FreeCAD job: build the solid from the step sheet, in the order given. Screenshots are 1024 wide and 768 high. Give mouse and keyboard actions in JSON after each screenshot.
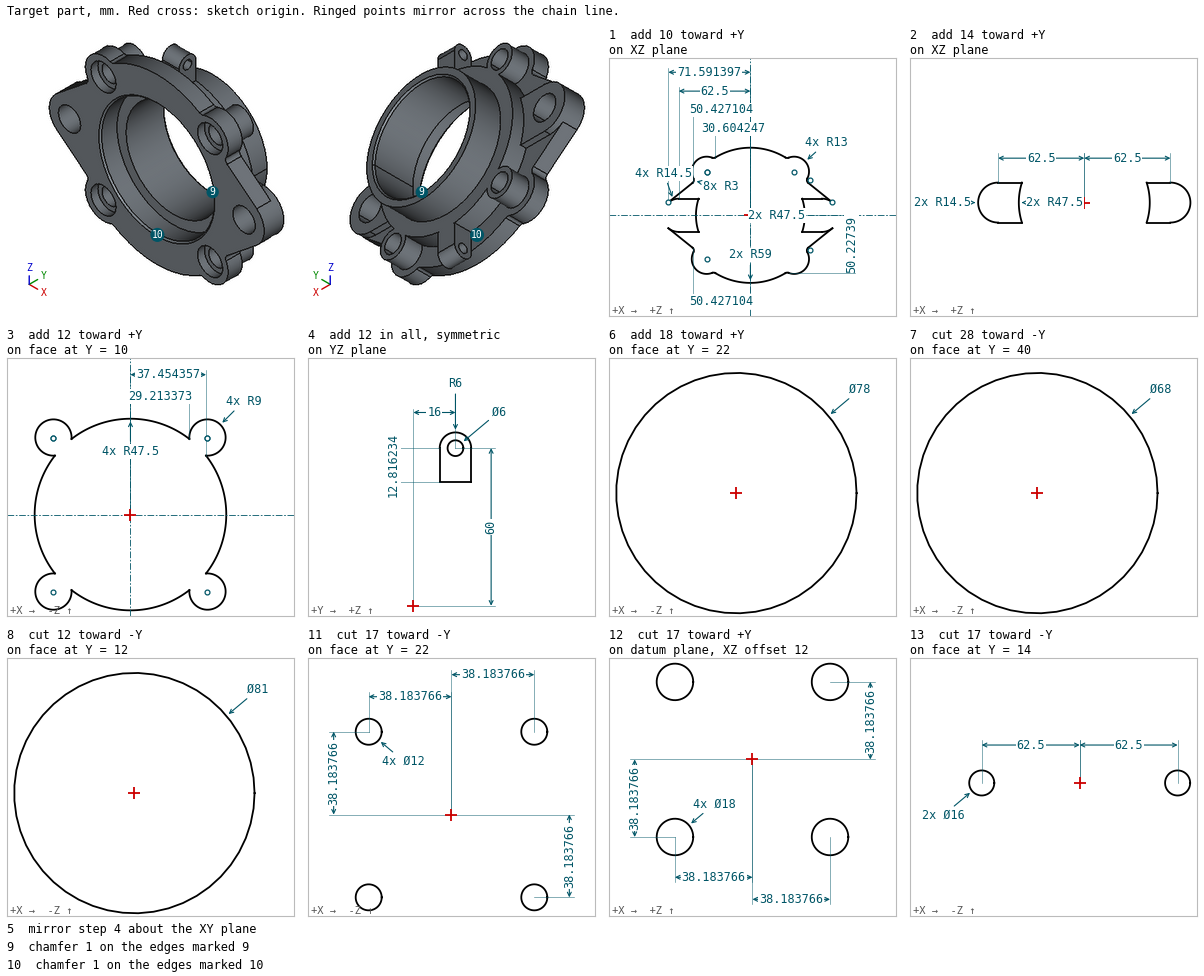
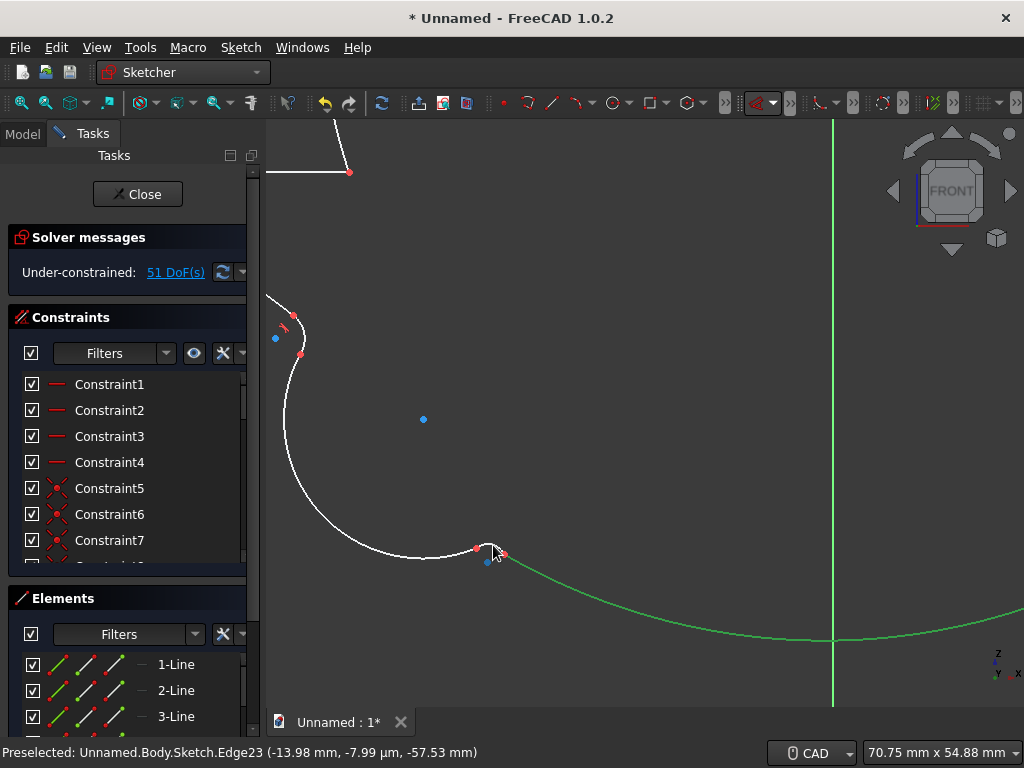
{"action": "left_click", "coordinate": [492, 545]}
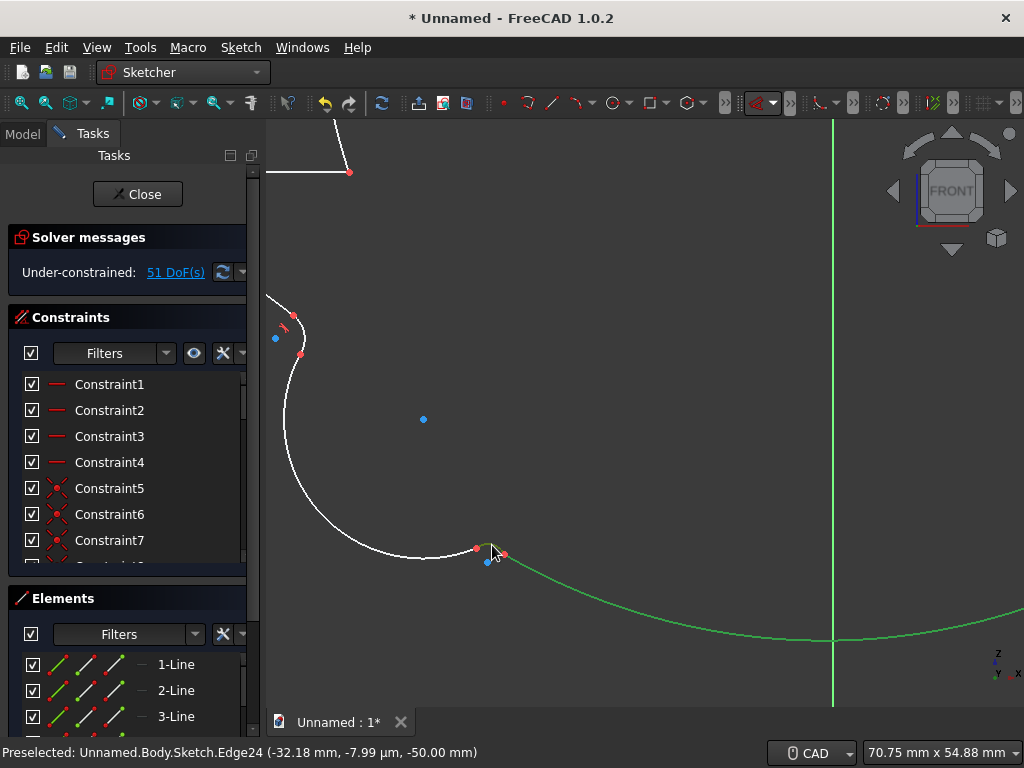
{"action": "key", "text": "t"}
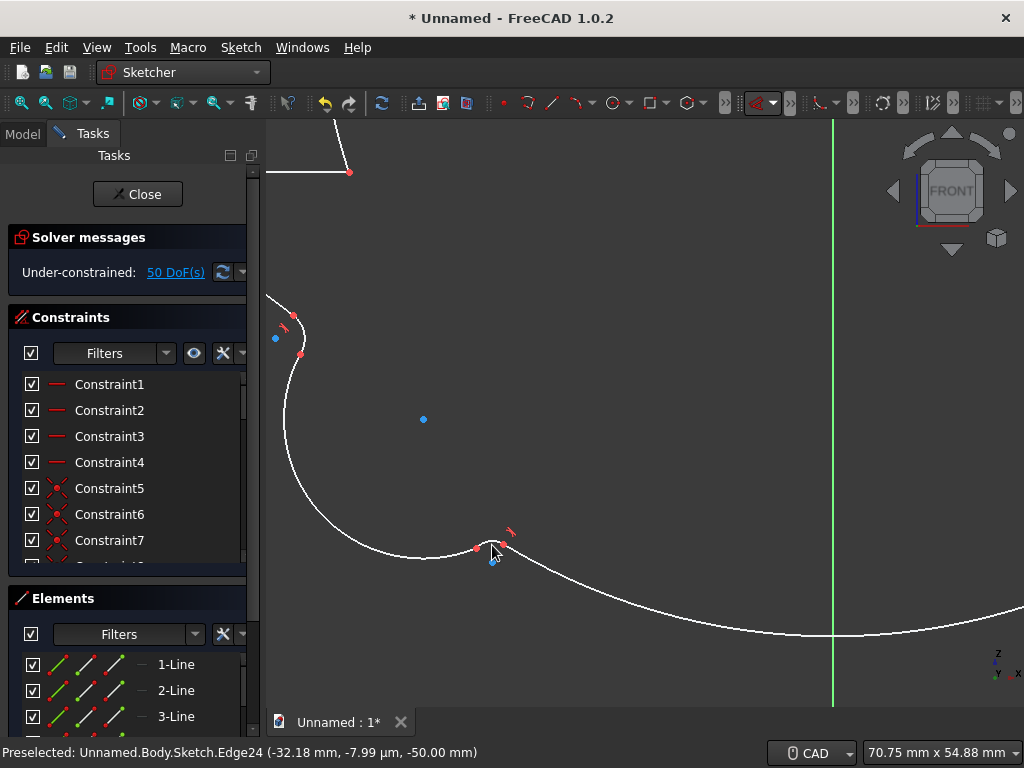
{"action": "left_click", "coordinate": [489, 541]}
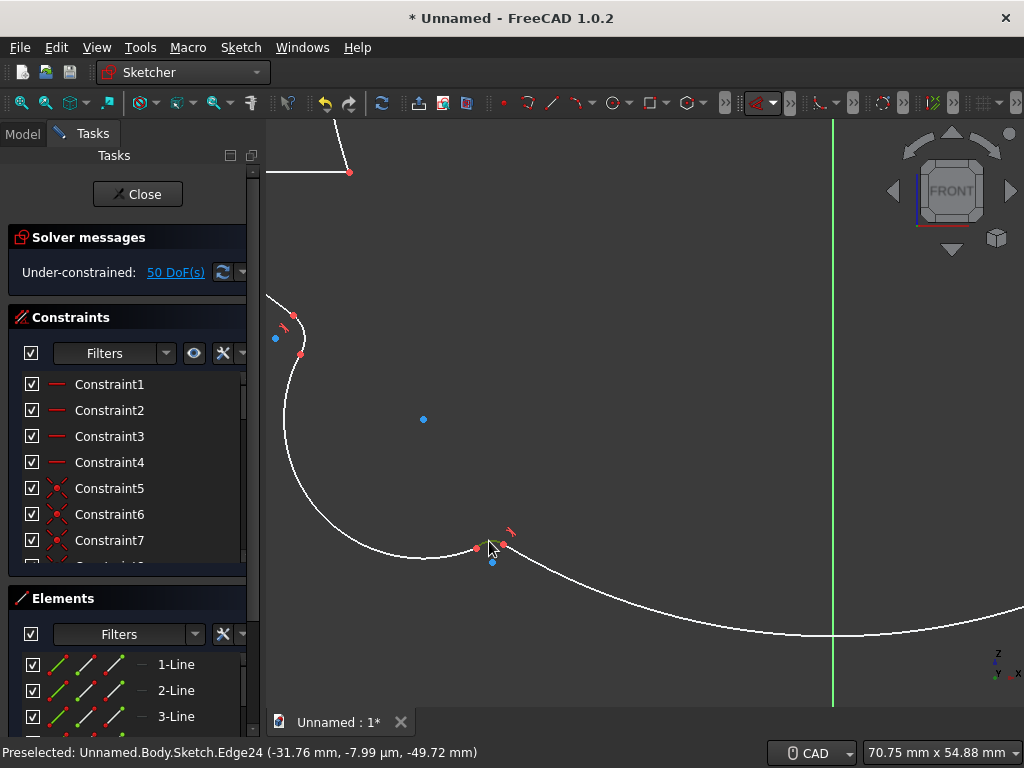
{"action": "scroll", "coordinate": [493, 545], "scroll_direction": "down", "scroll_amount": 7}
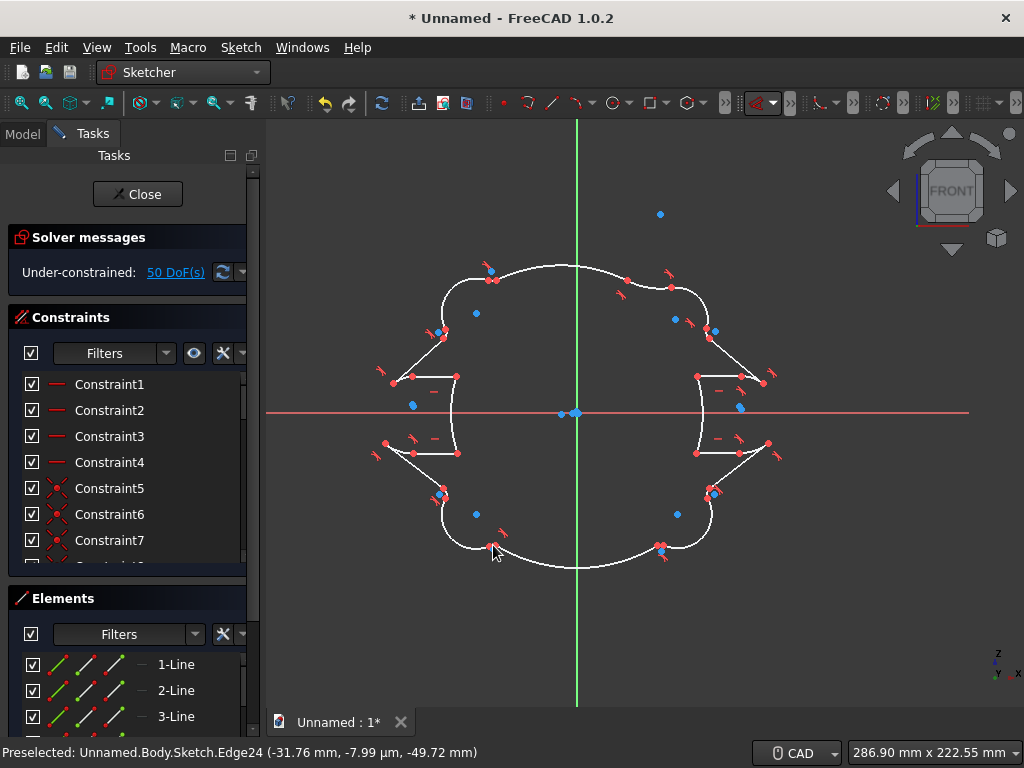
{"action": "left_click", "coordinate": [464, 547]}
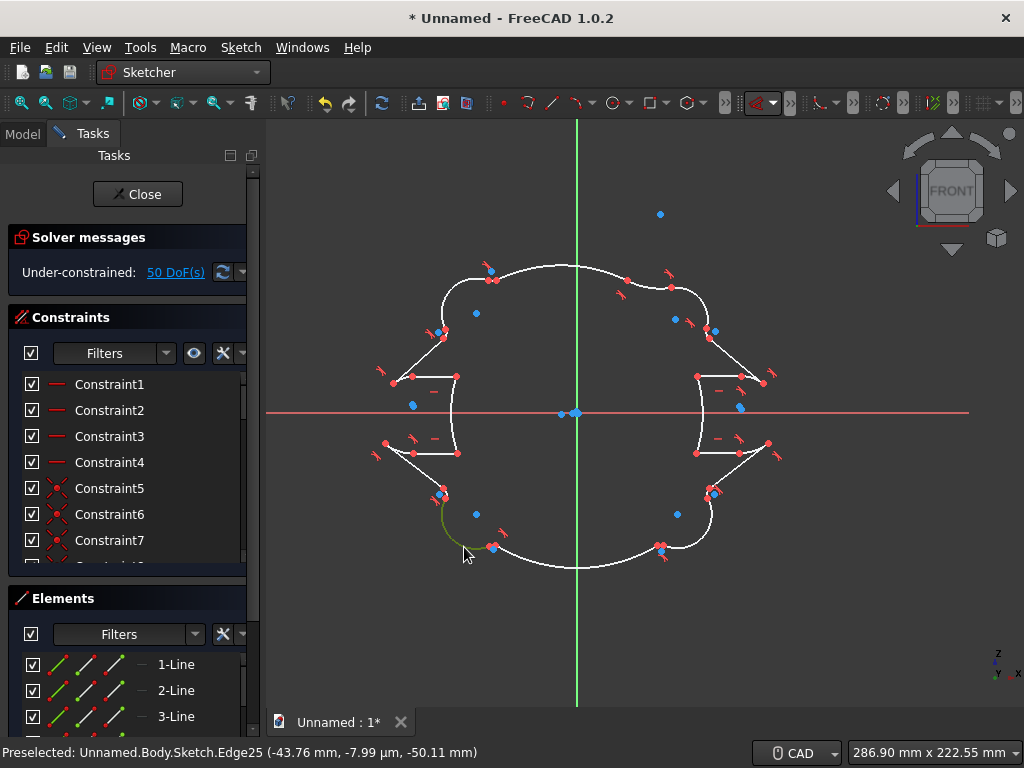
{"action": "key", "text": "t"}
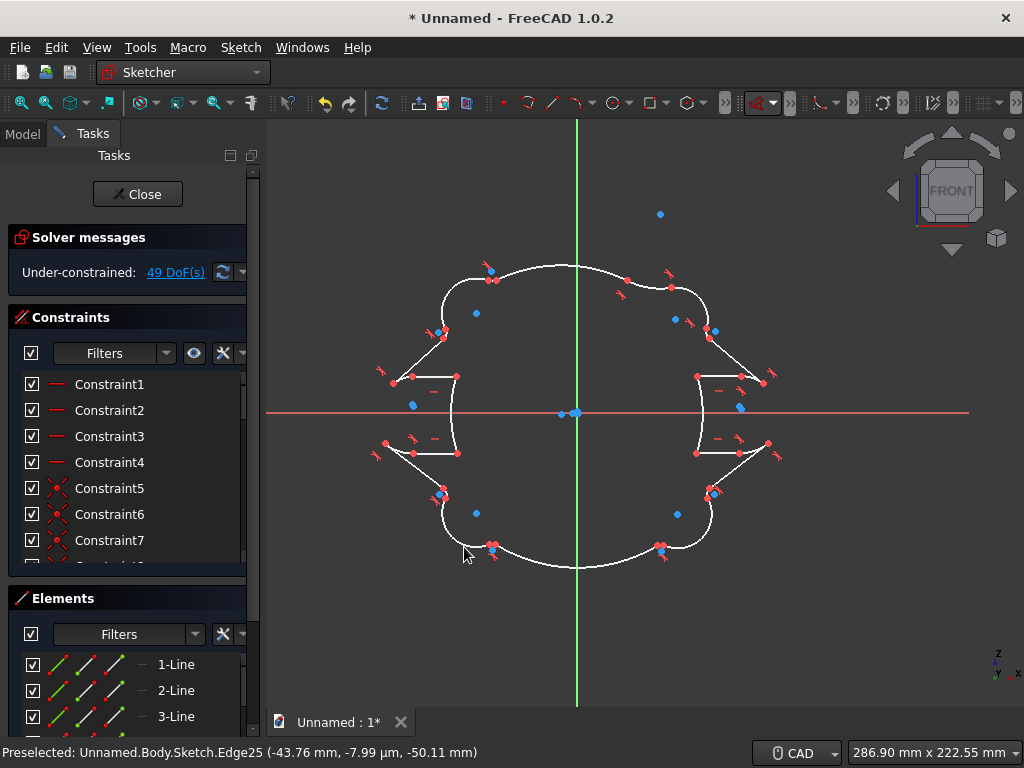
{"action": "left_click", "coordinate": [444, 523]}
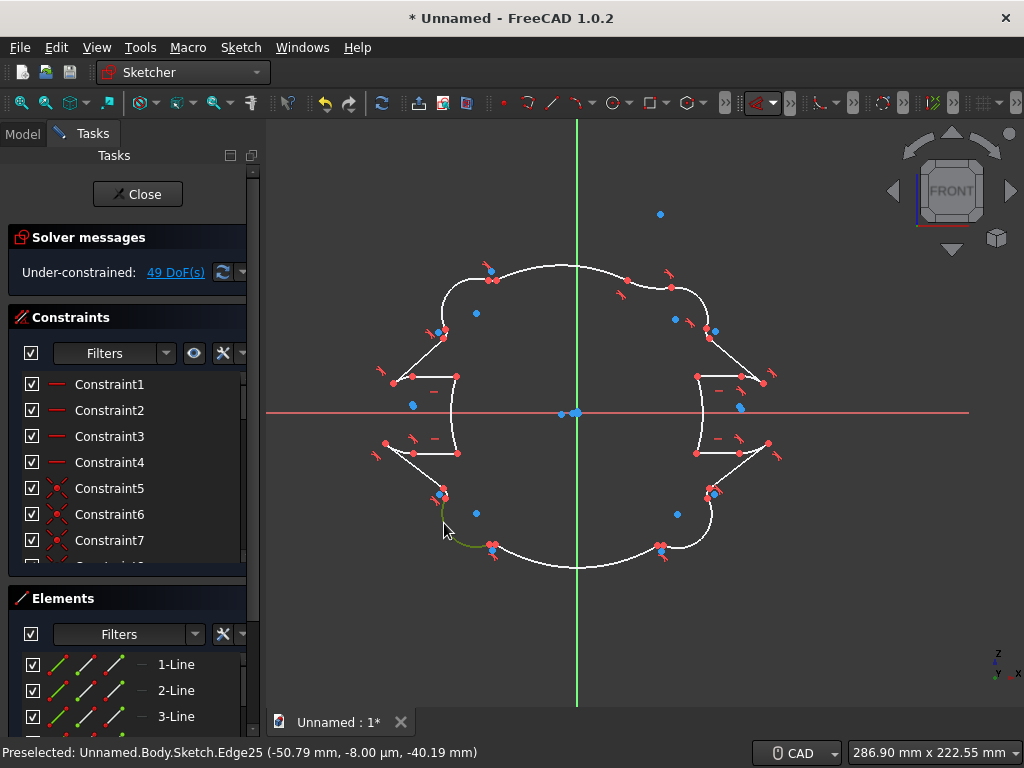
{"action": "scroll", "coordinate": [447, 493], "scroll_direction": "up", "scroll_amount": 5}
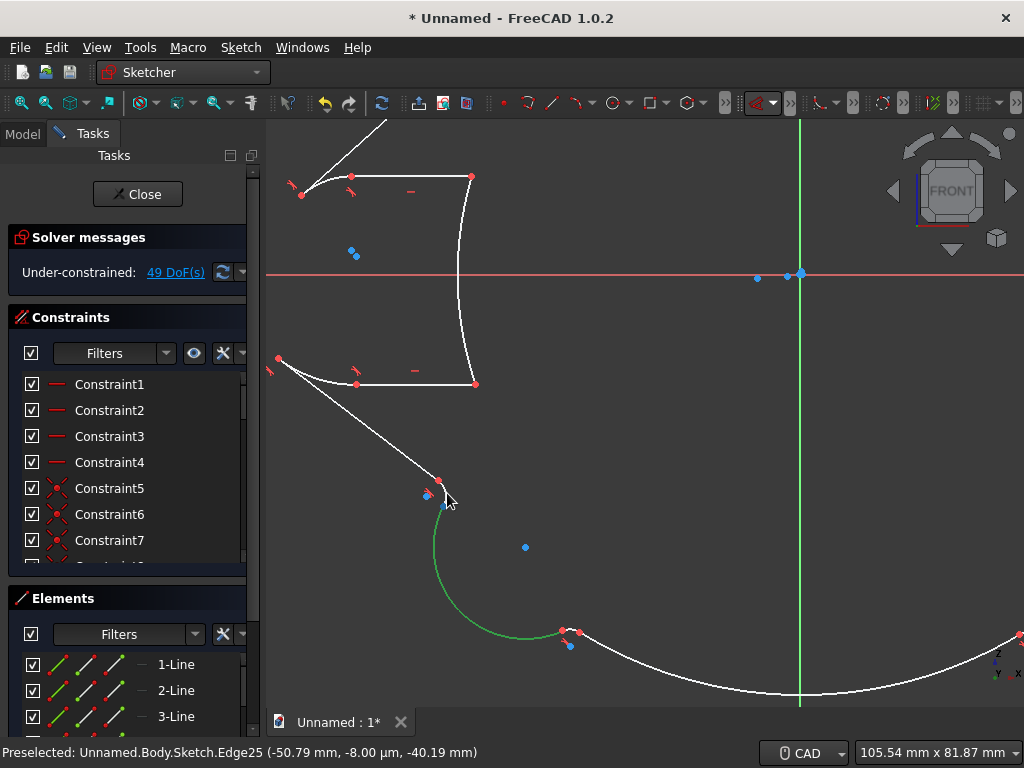
{"action": "left_click", "coordinate": [446, 493]}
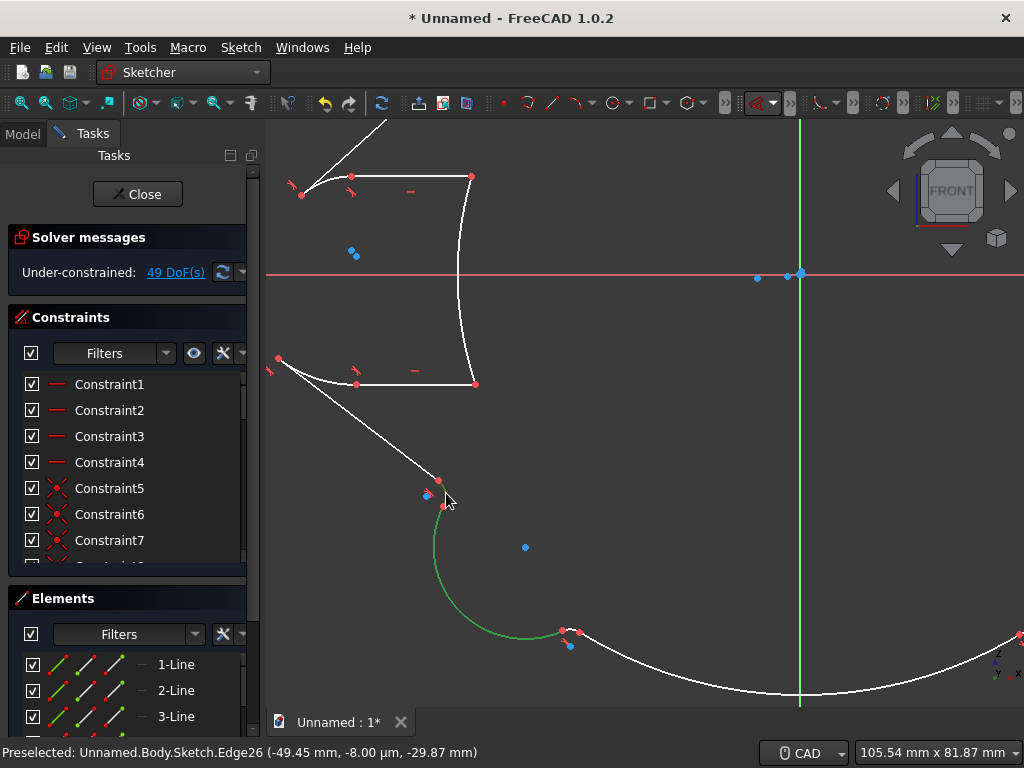
{"action": "key", "text": "t"}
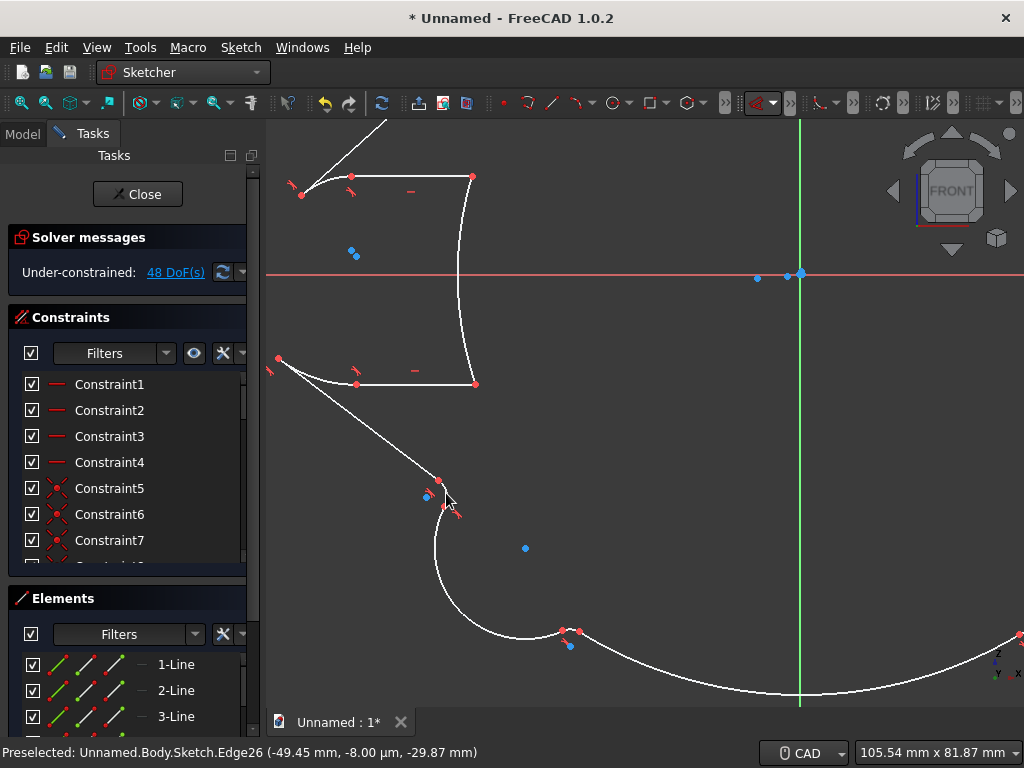
{"action": "scroll", "coordinate": [446, 493], "scroll_direction": "down", "scroll_amount": 5}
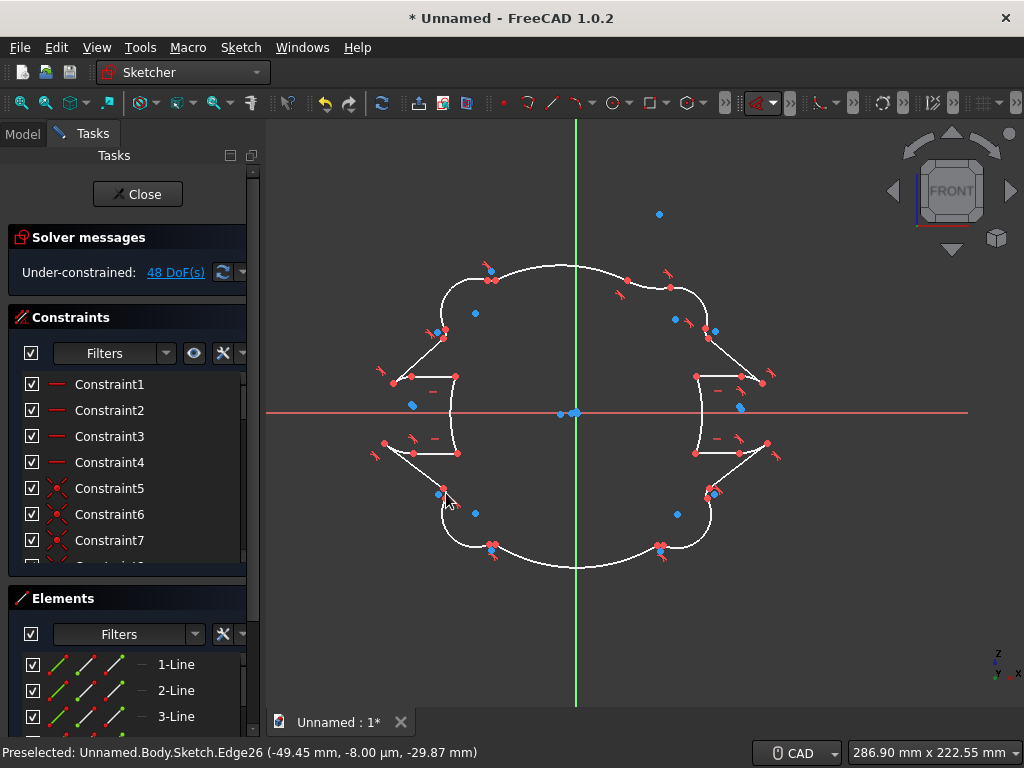
{"action": "left_click", "coordinate": [588, 268]}